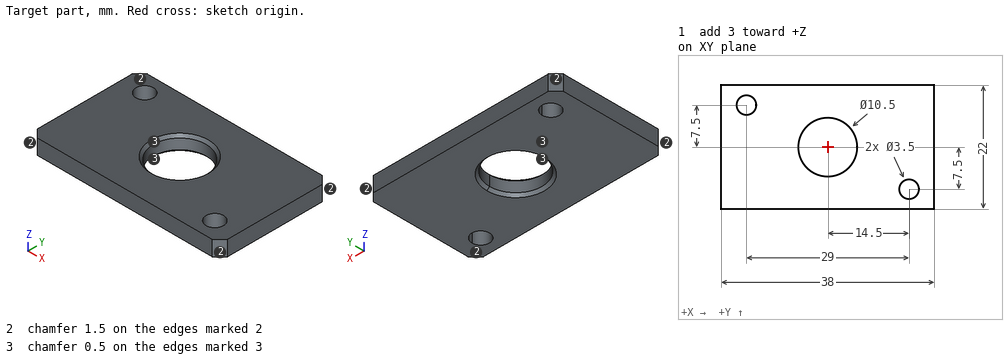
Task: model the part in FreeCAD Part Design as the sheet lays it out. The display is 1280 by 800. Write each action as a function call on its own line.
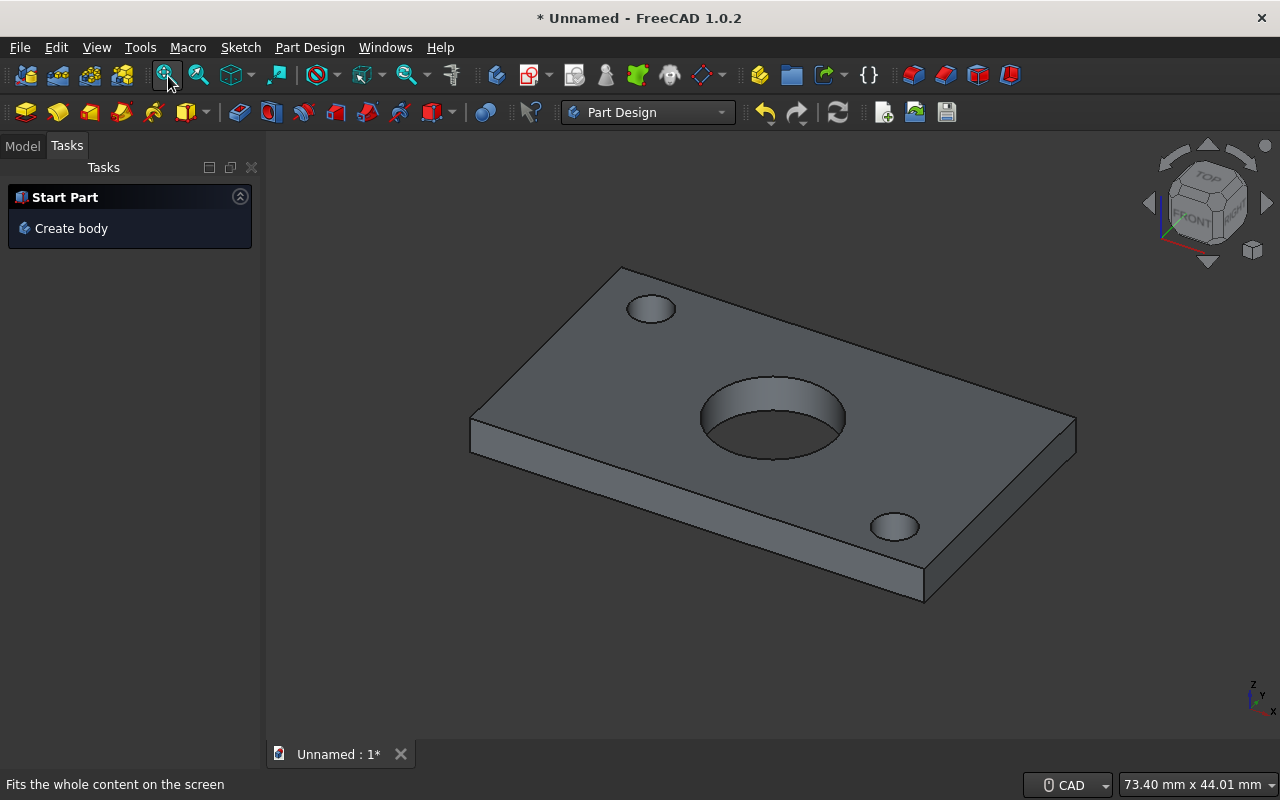
click(924, 585)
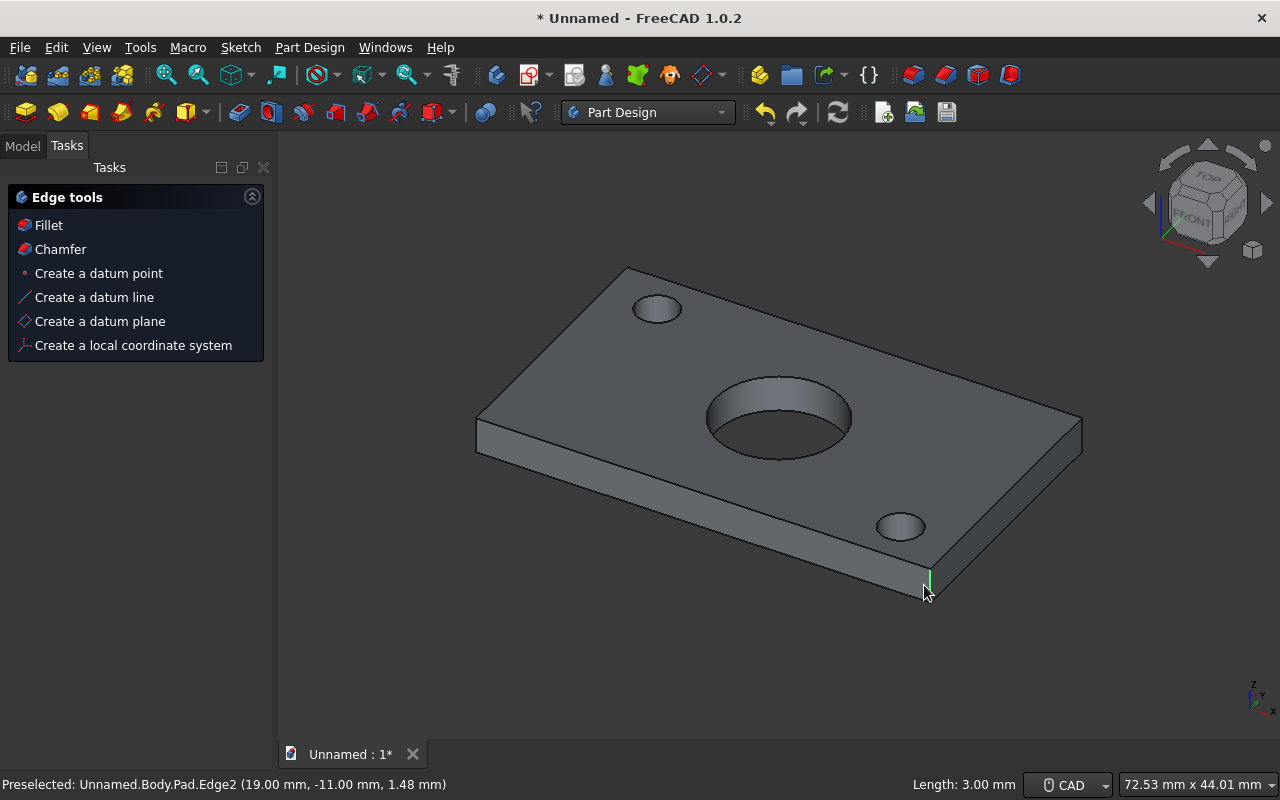
key(0)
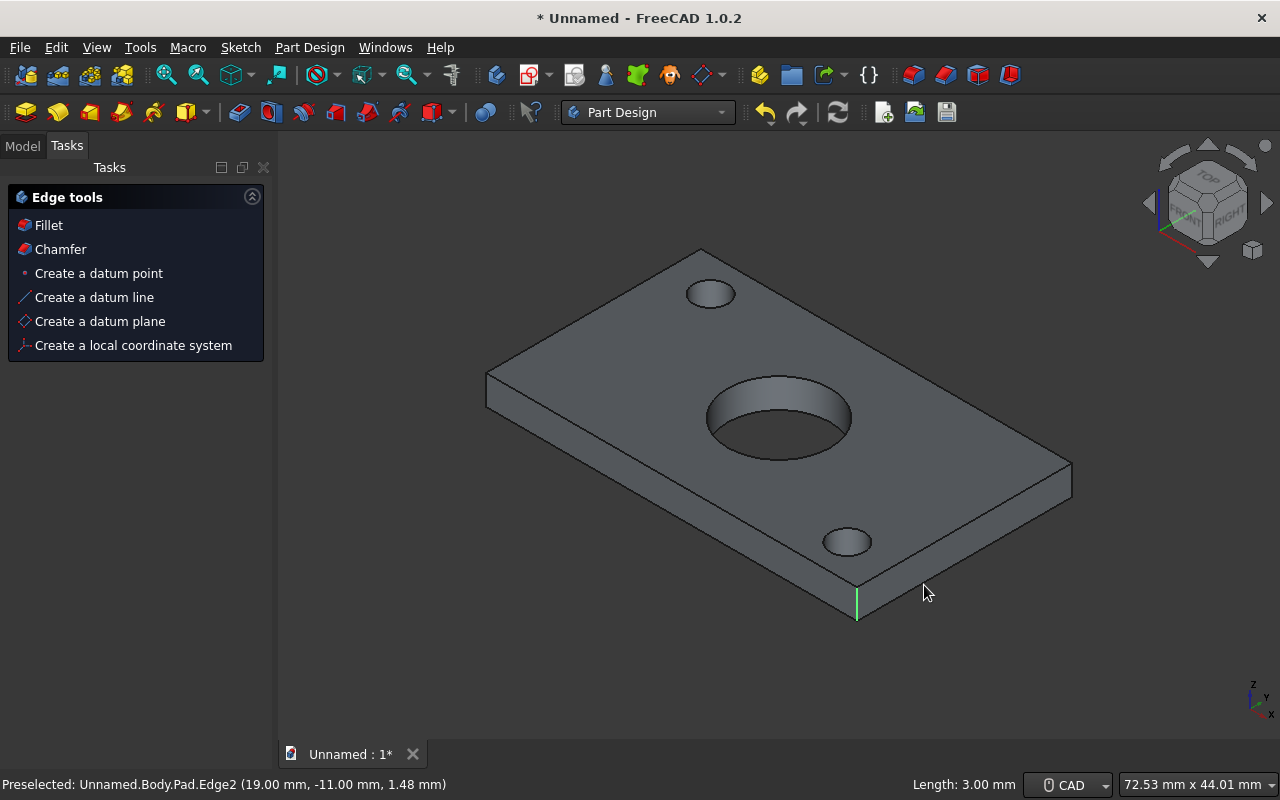
key(2)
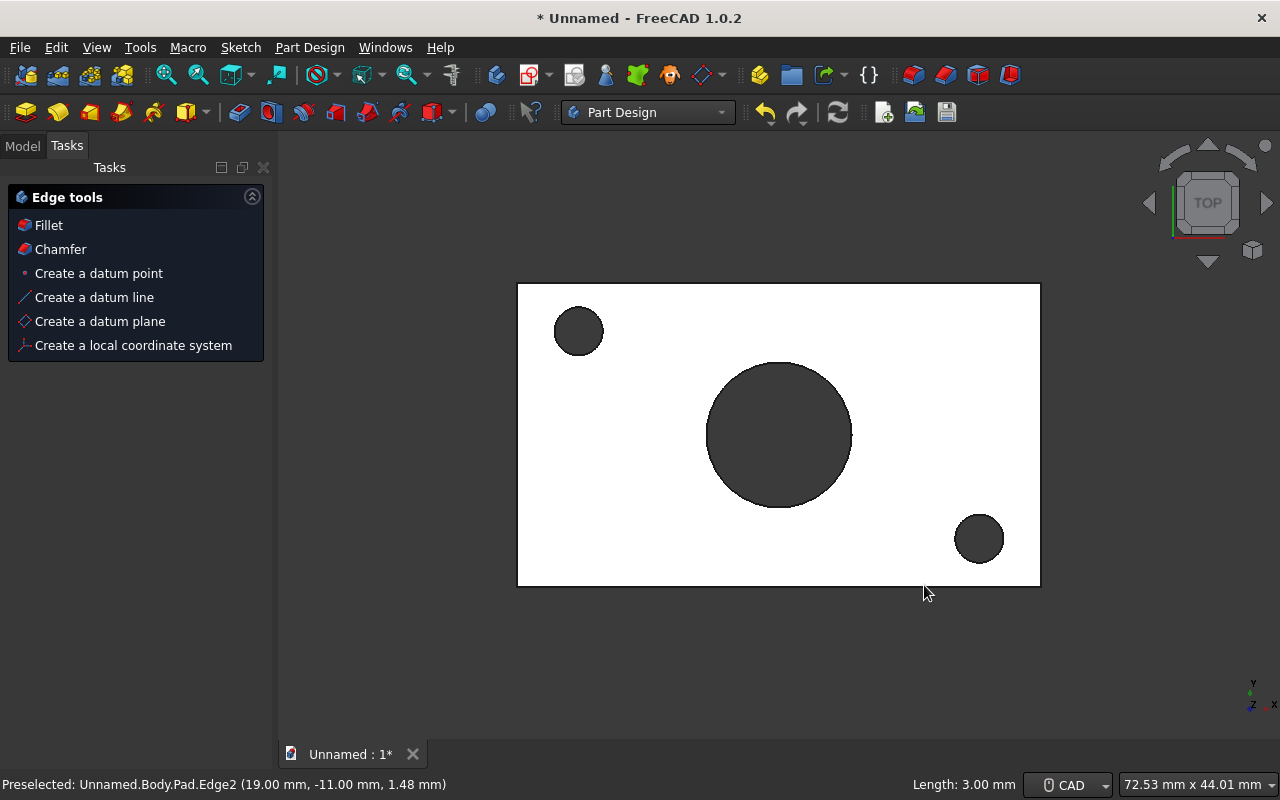
key(1)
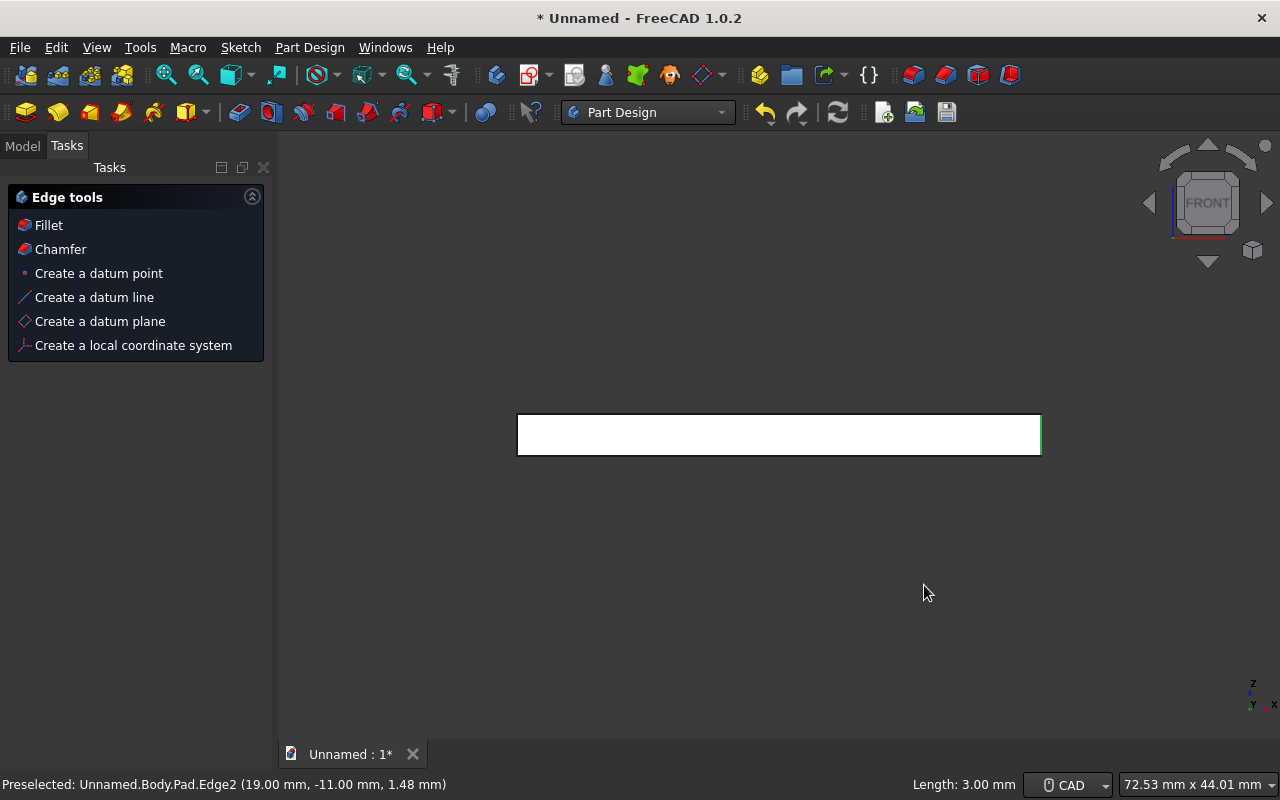
click(517, 434, ctrl)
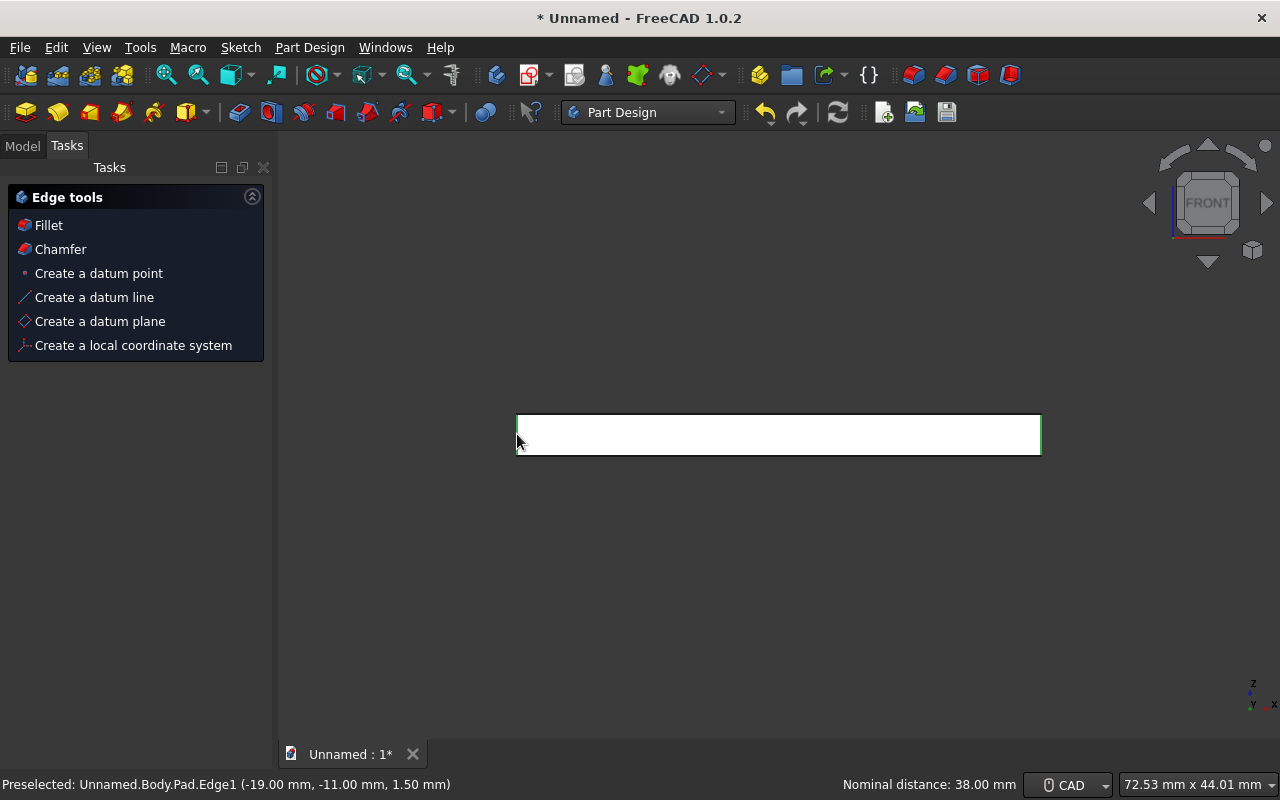
key(3)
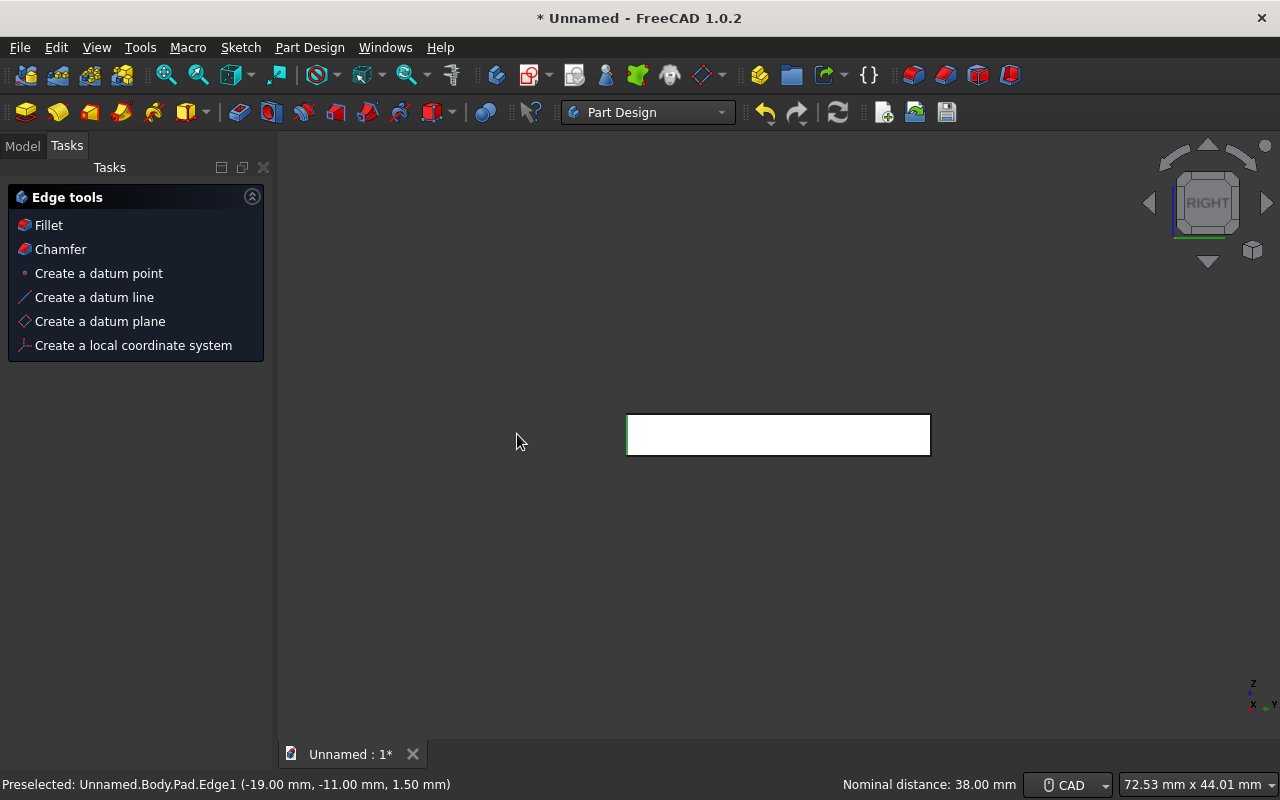
click(168, 76)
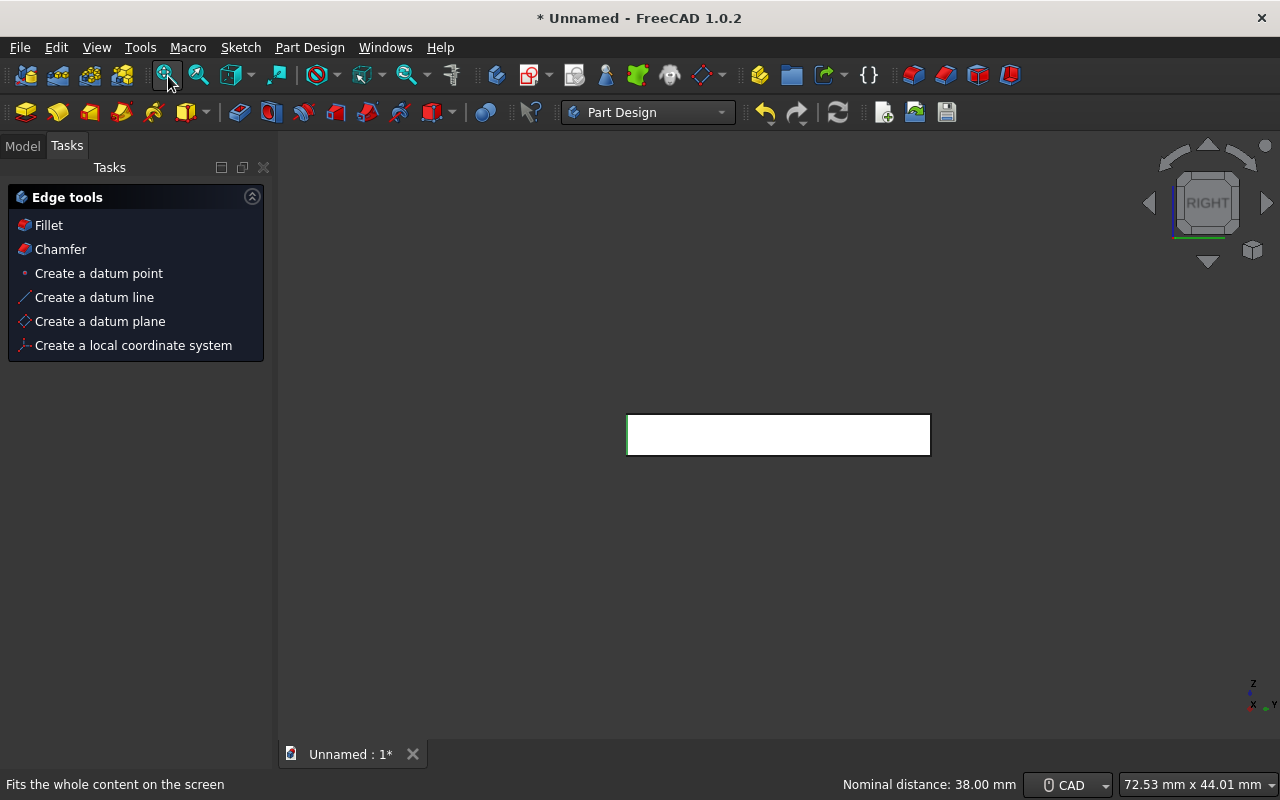
click(931, 434, ctrl)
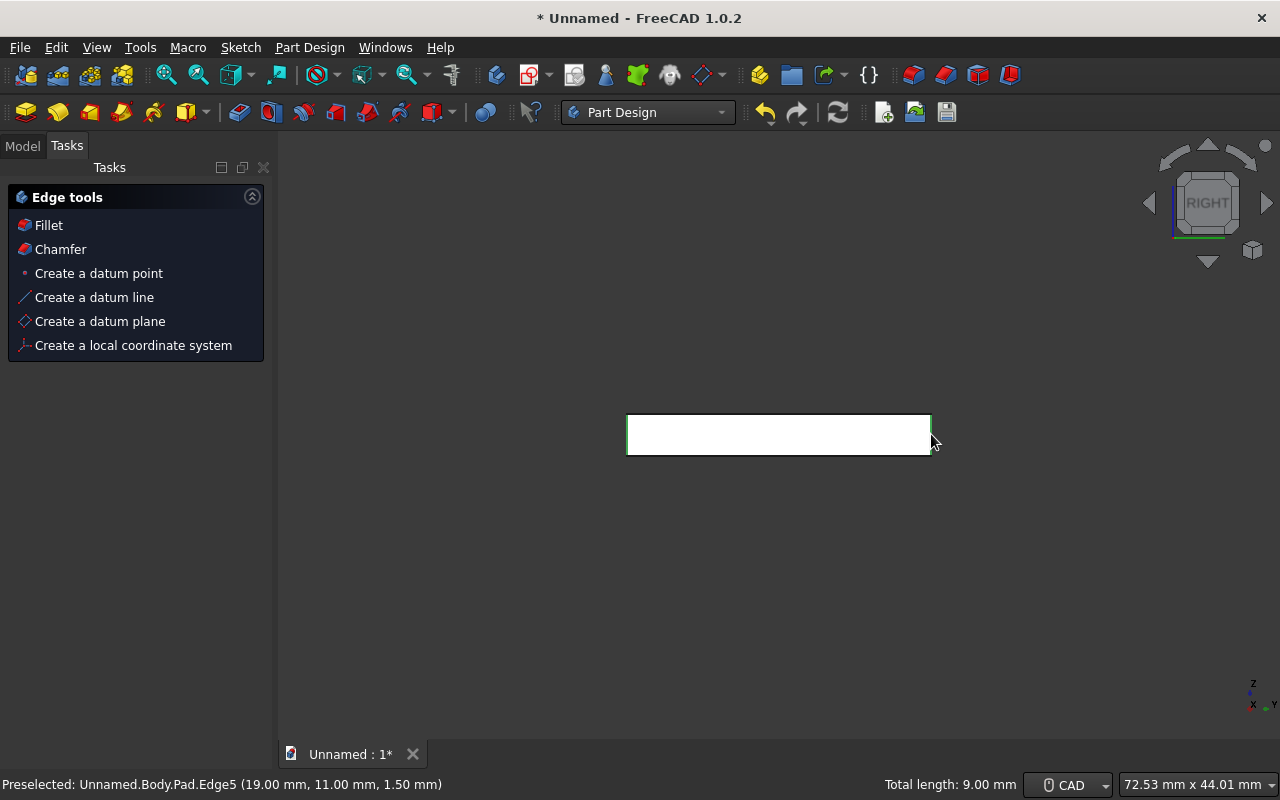
key(5)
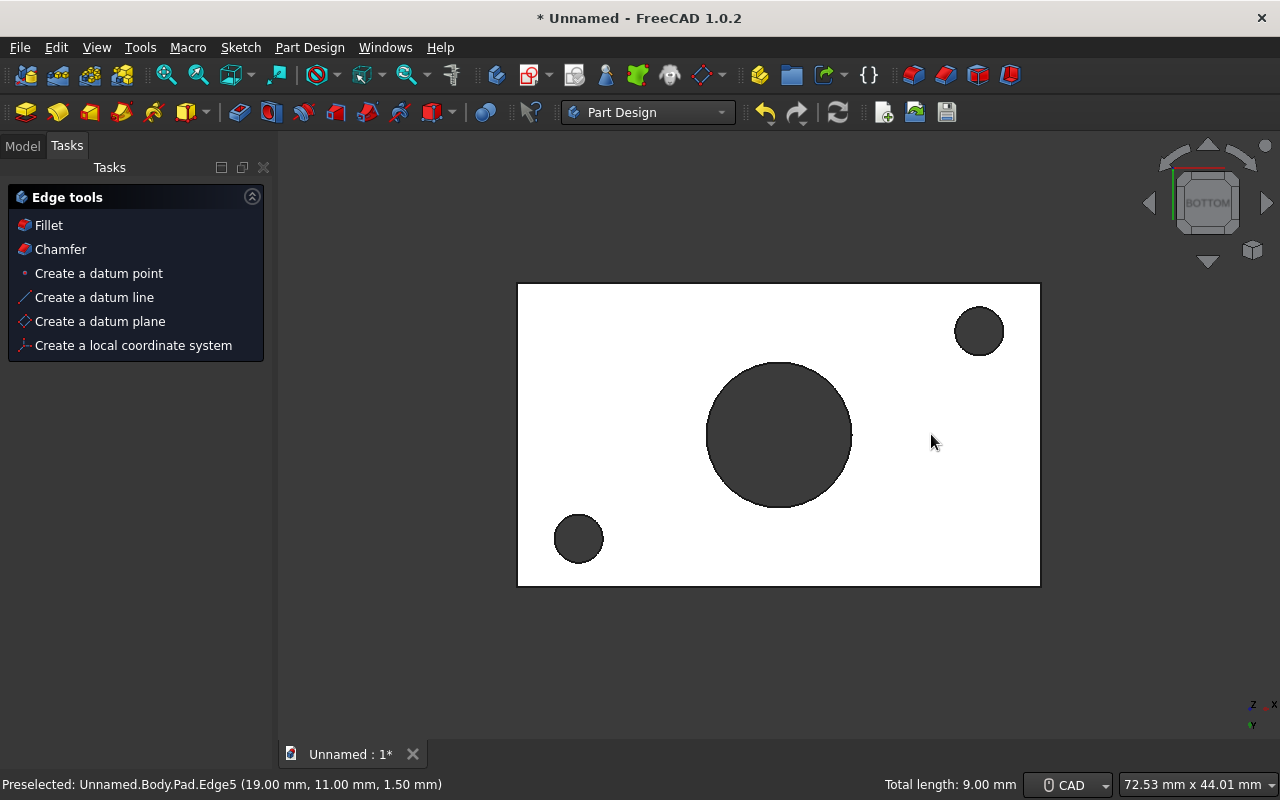
key(4)